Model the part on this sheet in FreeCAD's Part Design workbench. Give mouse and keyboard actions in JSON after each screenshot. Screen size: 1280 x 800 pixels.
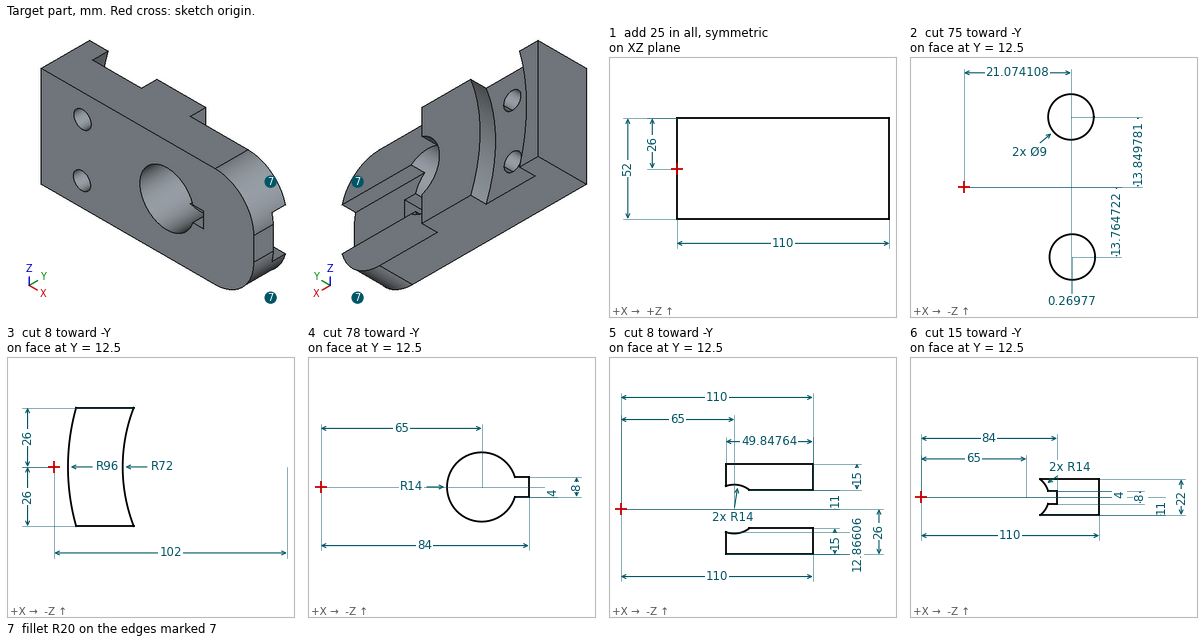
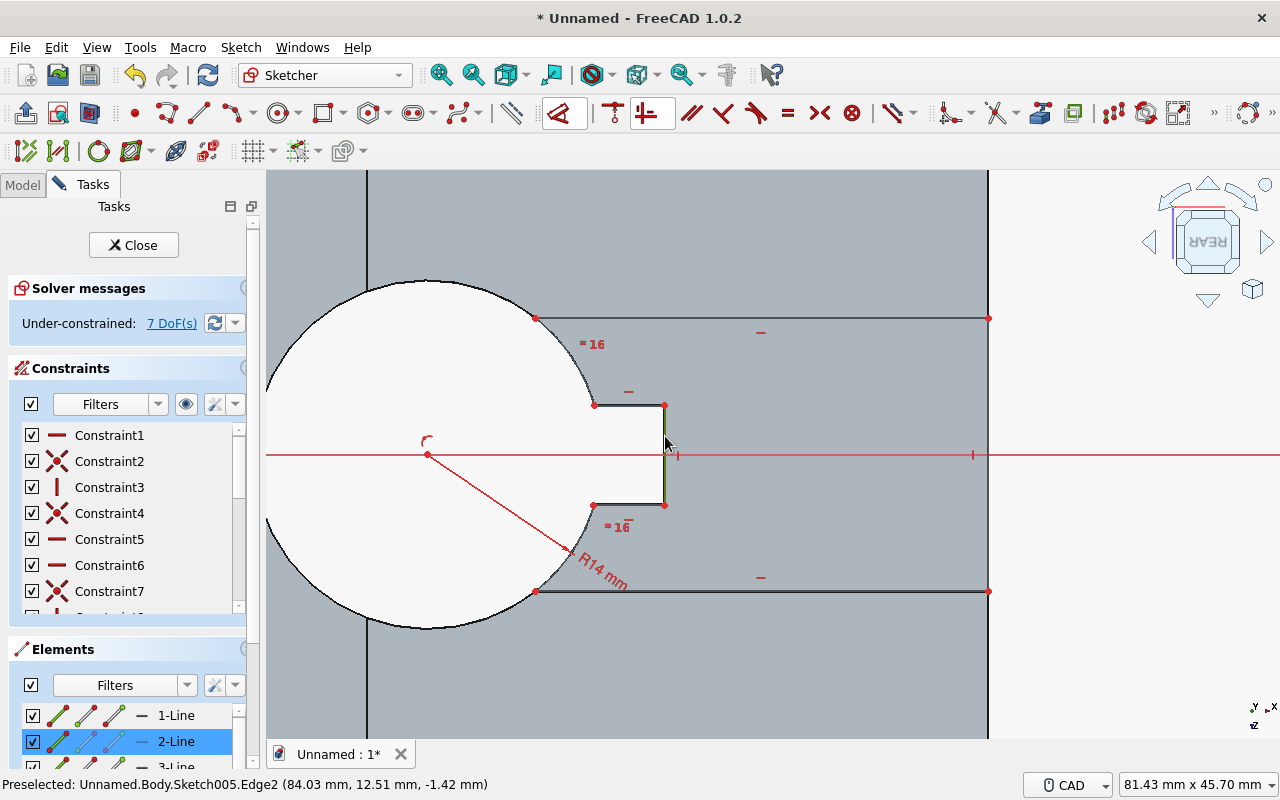
{"action": "left_click", "coordinate": [582, 114]}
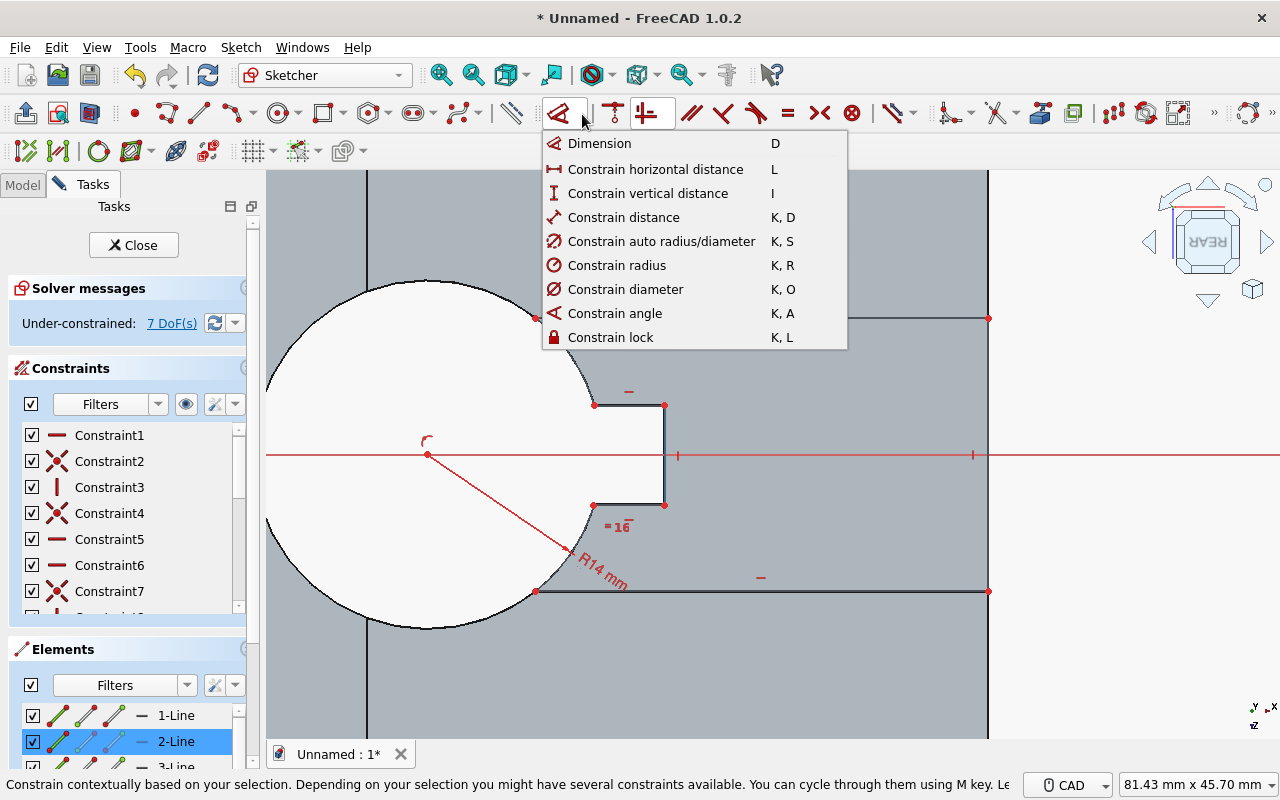
{"action": "left_click", "coordinate": [695, 193]}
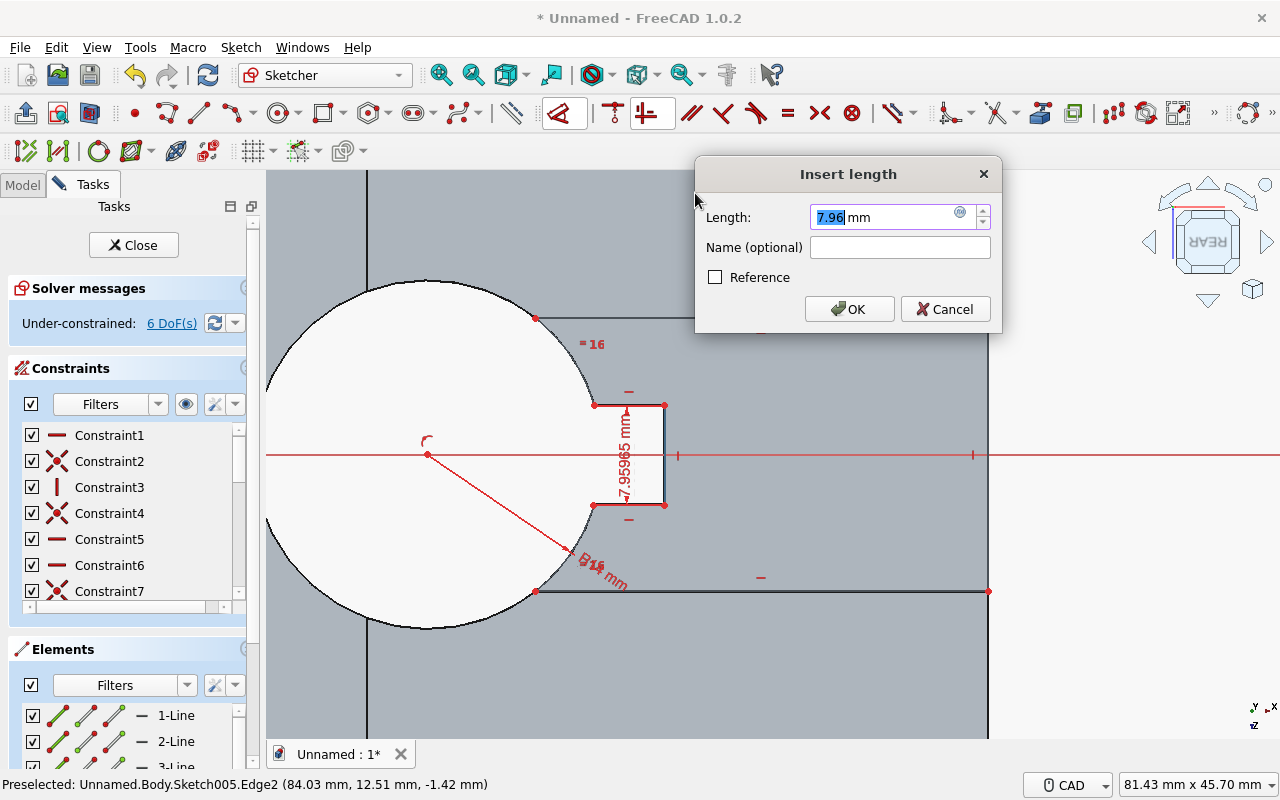
{"action": "type", "text": "8"}
{"action": "key", "text": "Return"}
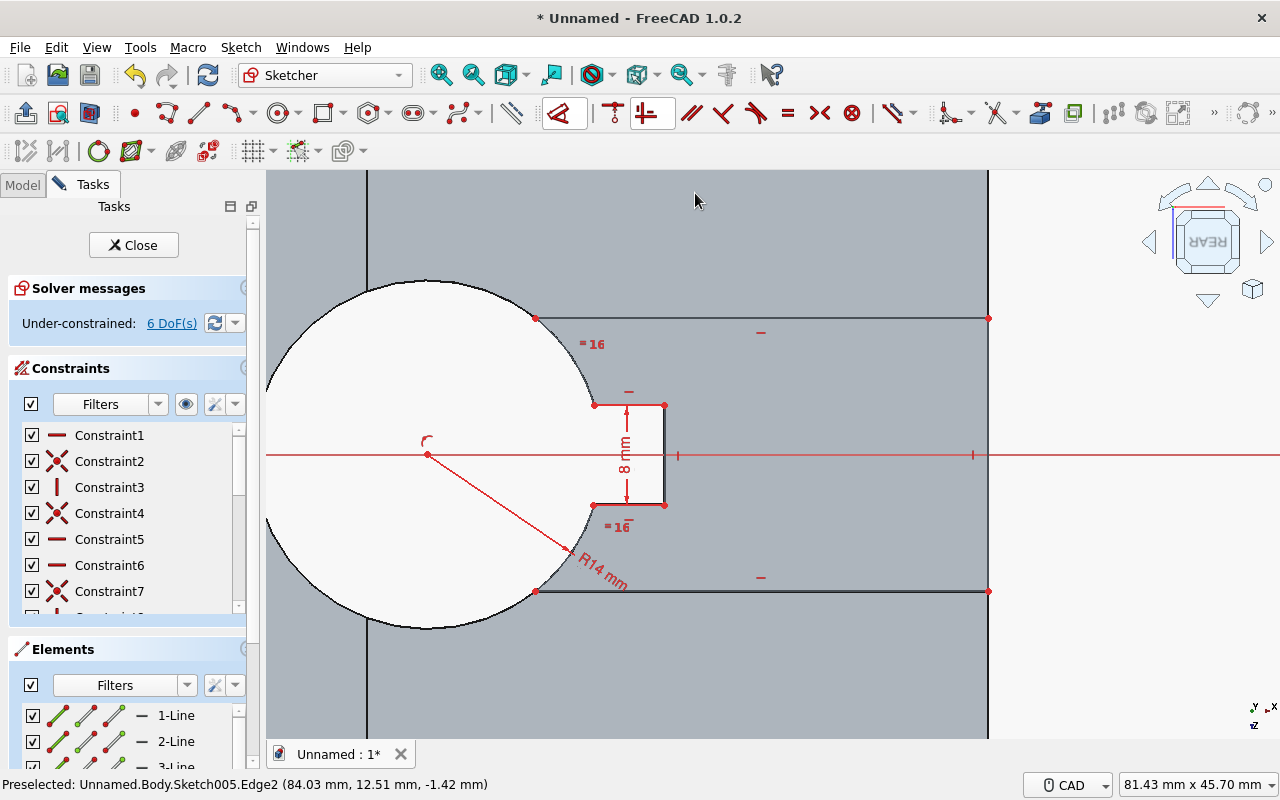
{"action": "left_click", "coordinate": [988, 509]}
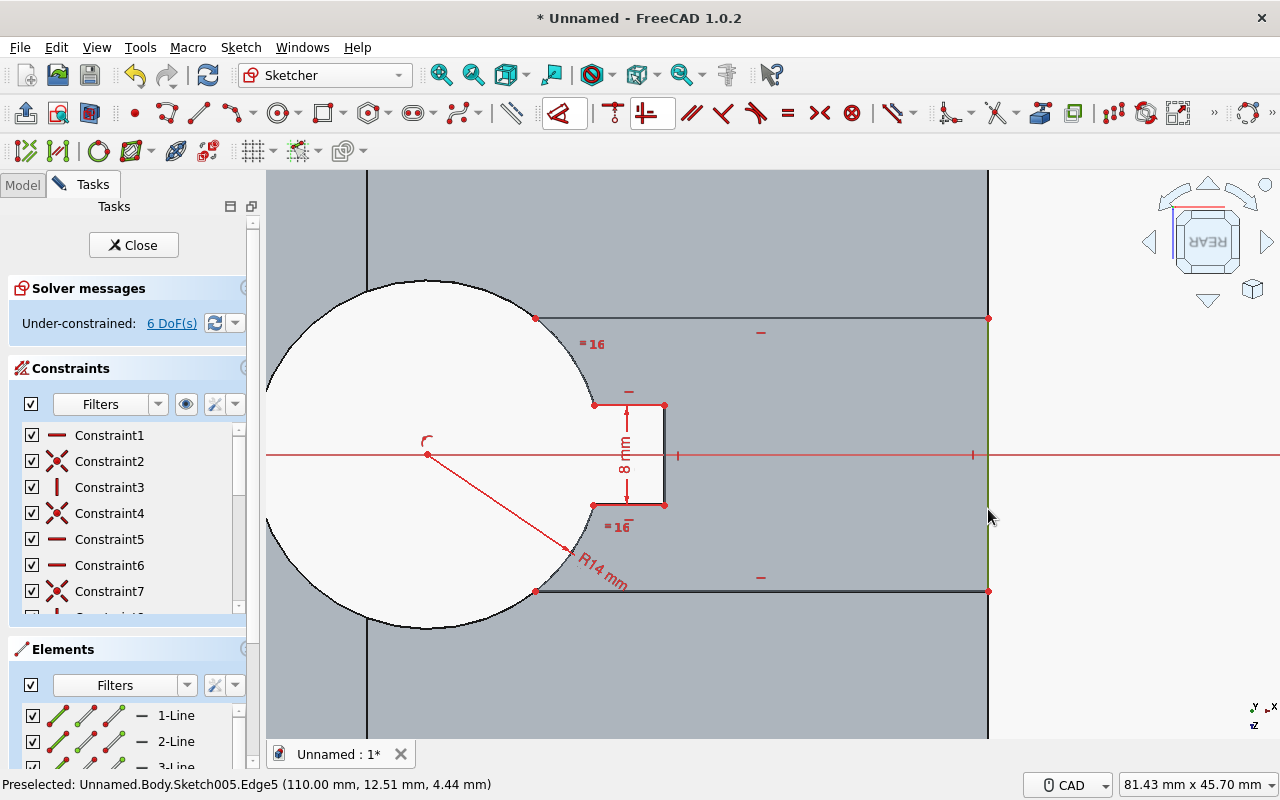
{"action": "key", "text": "i"}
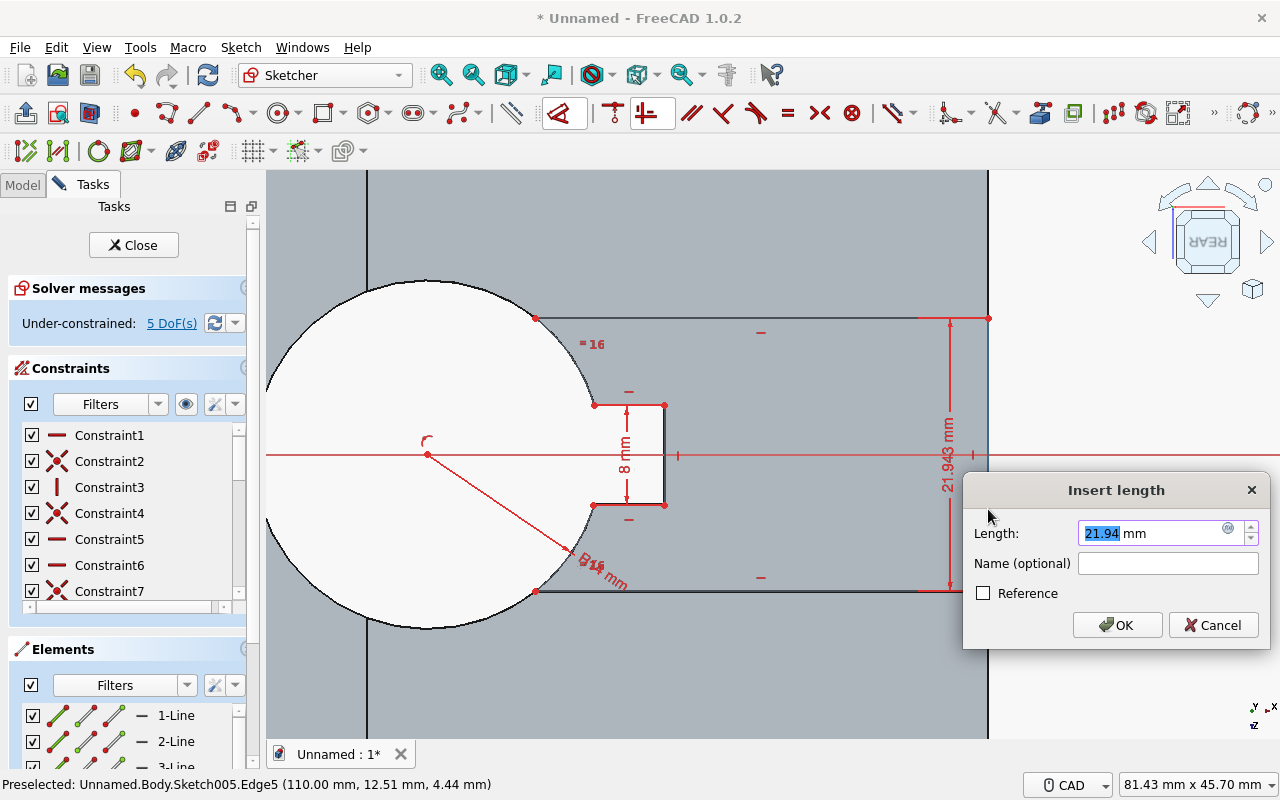
{"action": "type", "text": "22"}
{"action": "key", "text": "Return"}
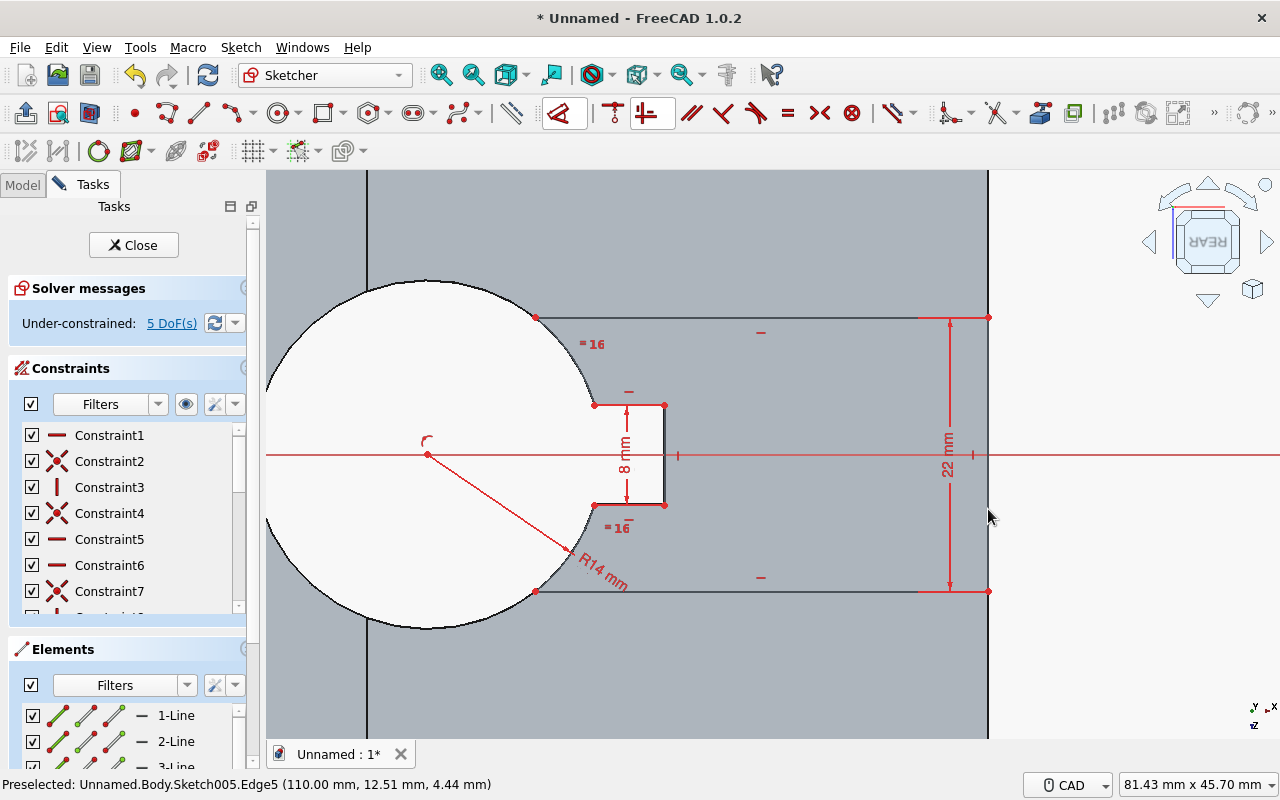
{"action": "left_click", "coordinate": [595, 405]}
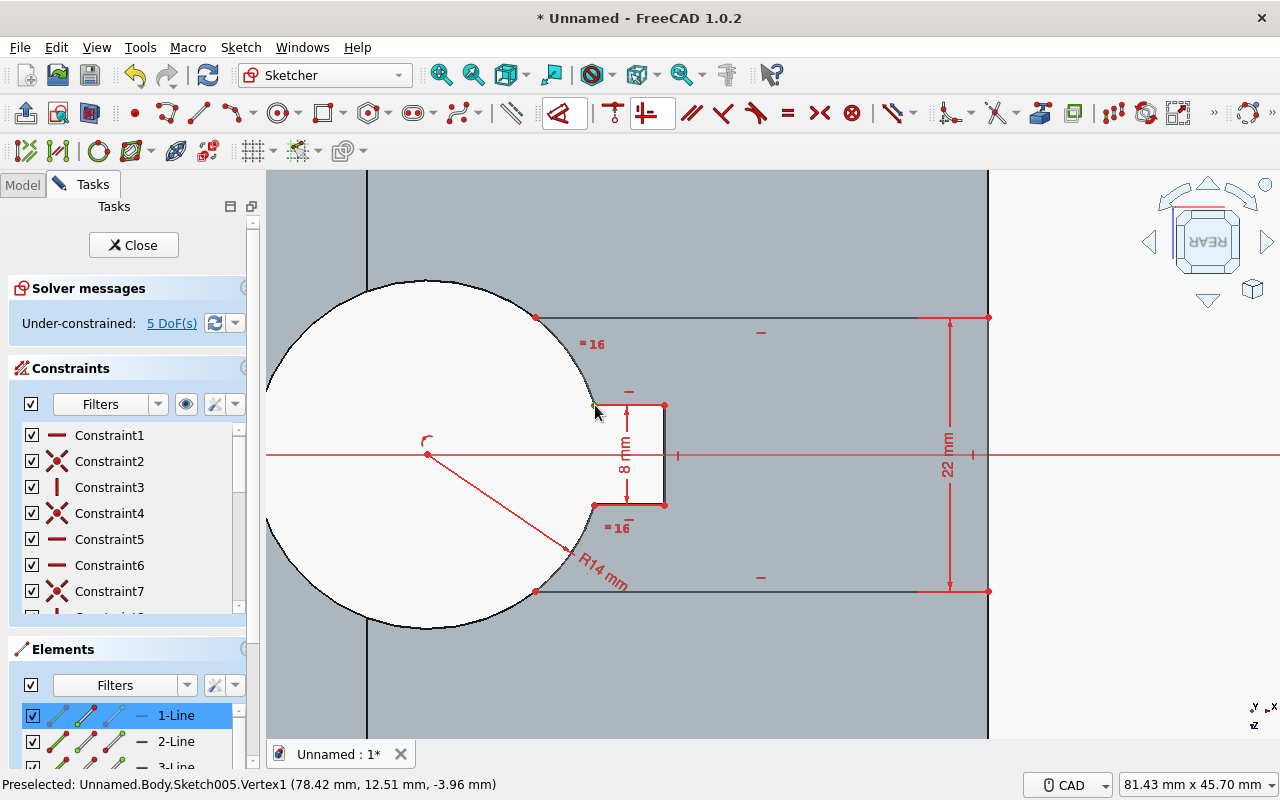
{"action": "left_click", "coordinate": [582, 114]}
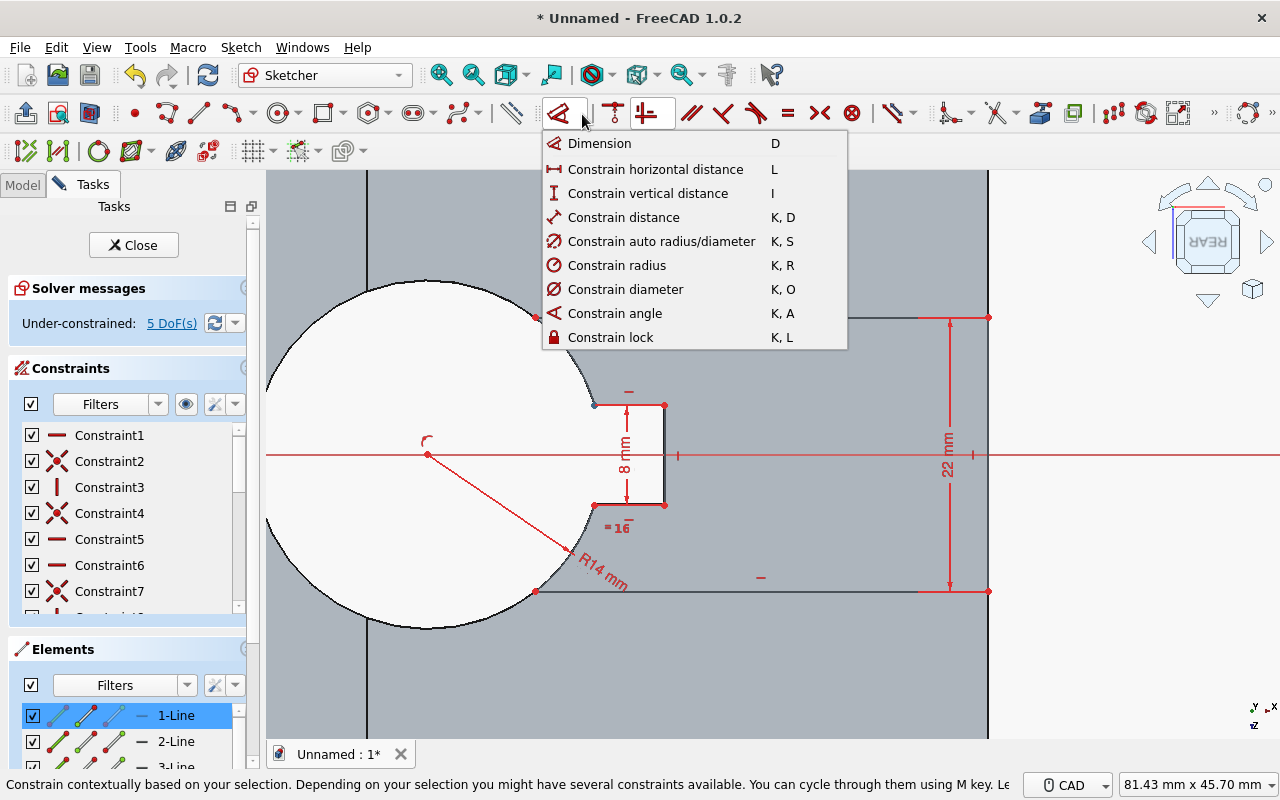
{"action": "left_click", "coordinate": [695, 193]}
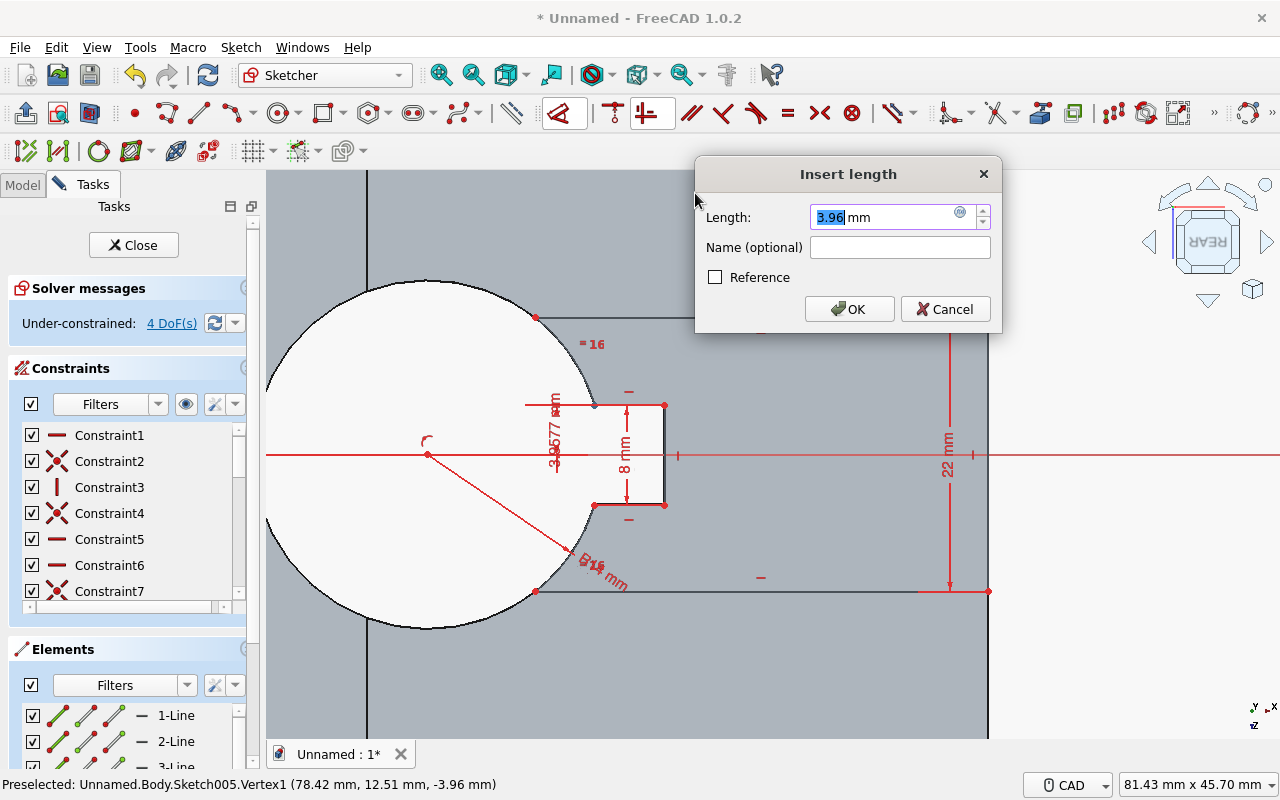
{"action": "type", "text": "4"}
{"action": "key", "text": "Return"}